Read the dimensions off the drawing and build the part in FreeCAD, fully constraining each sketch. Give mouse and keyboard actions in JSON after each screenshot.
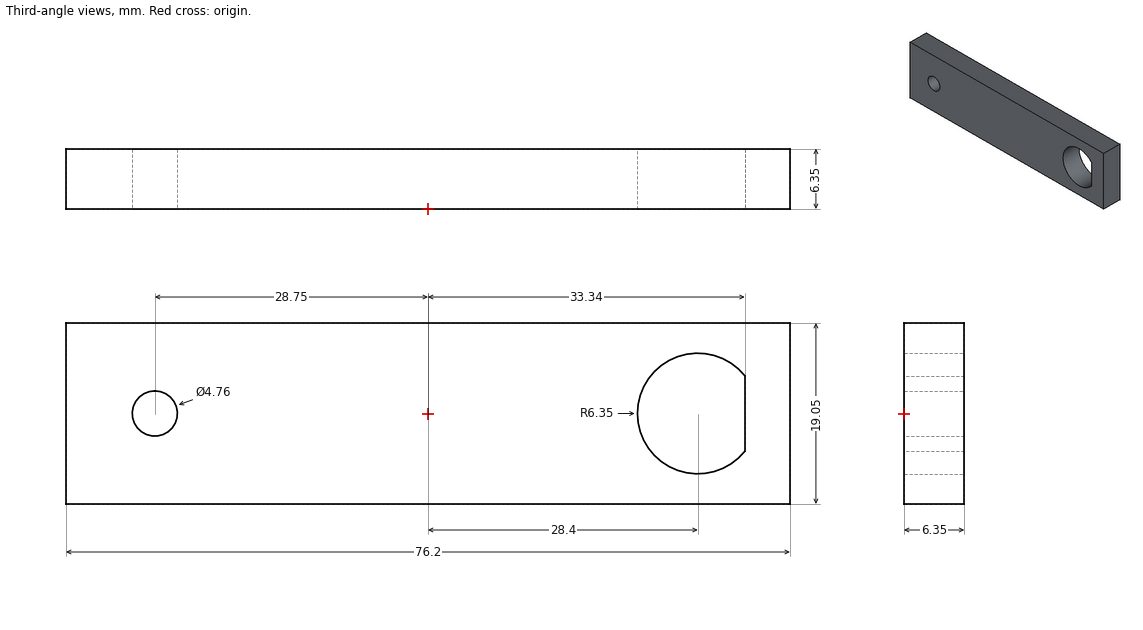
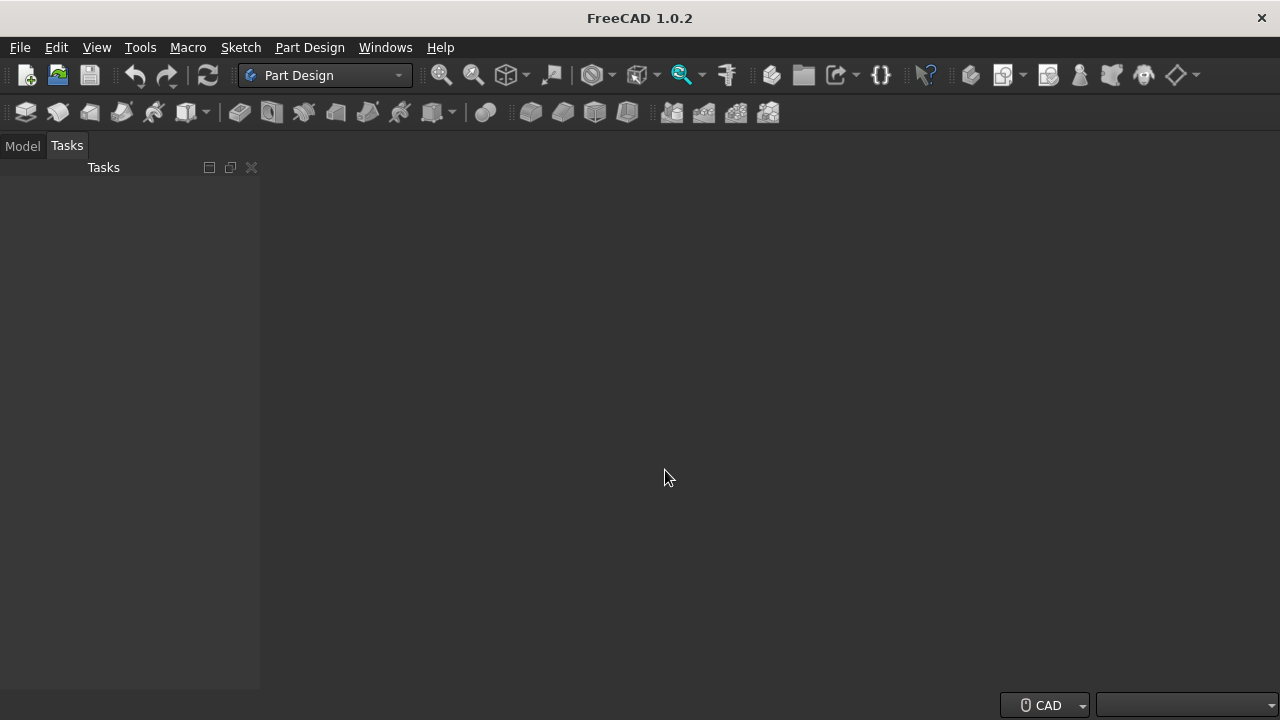
{"action": "key", "text": "ctrl+n"}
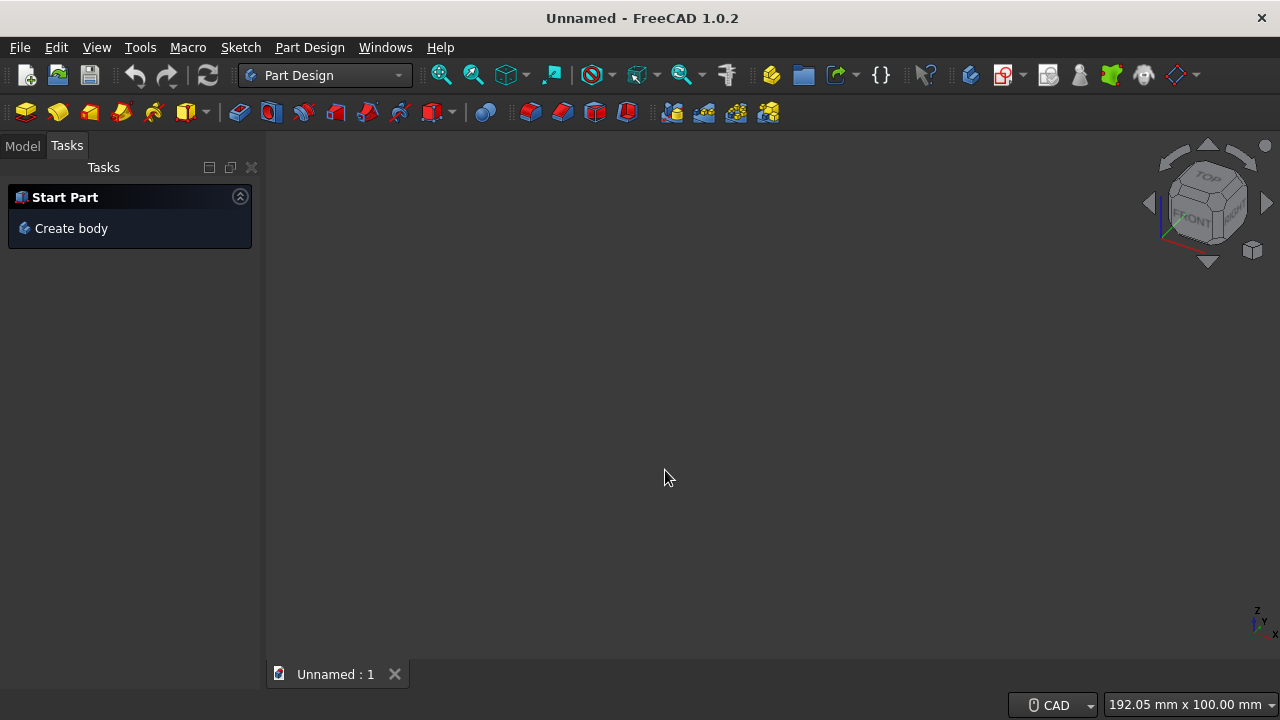
{"action": "left_click", "coordinate": [1004, 76]}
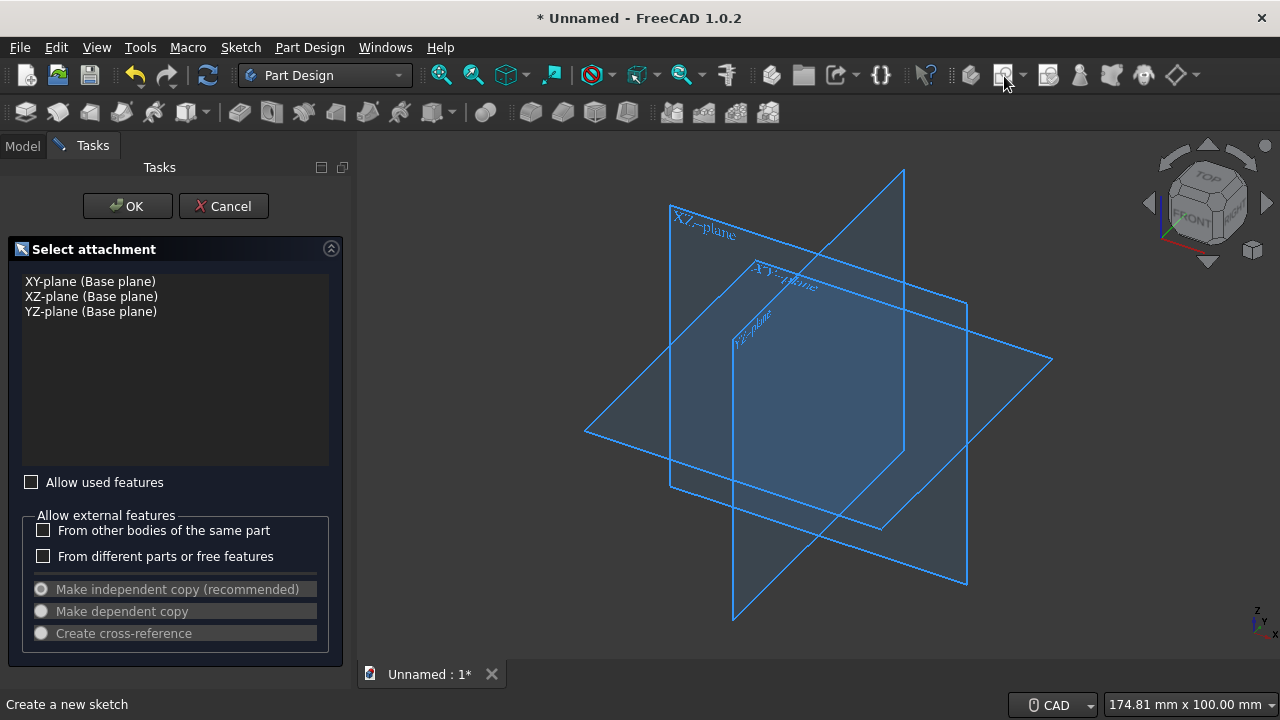
{"action": "left_click", "coordinate": [82, 296]}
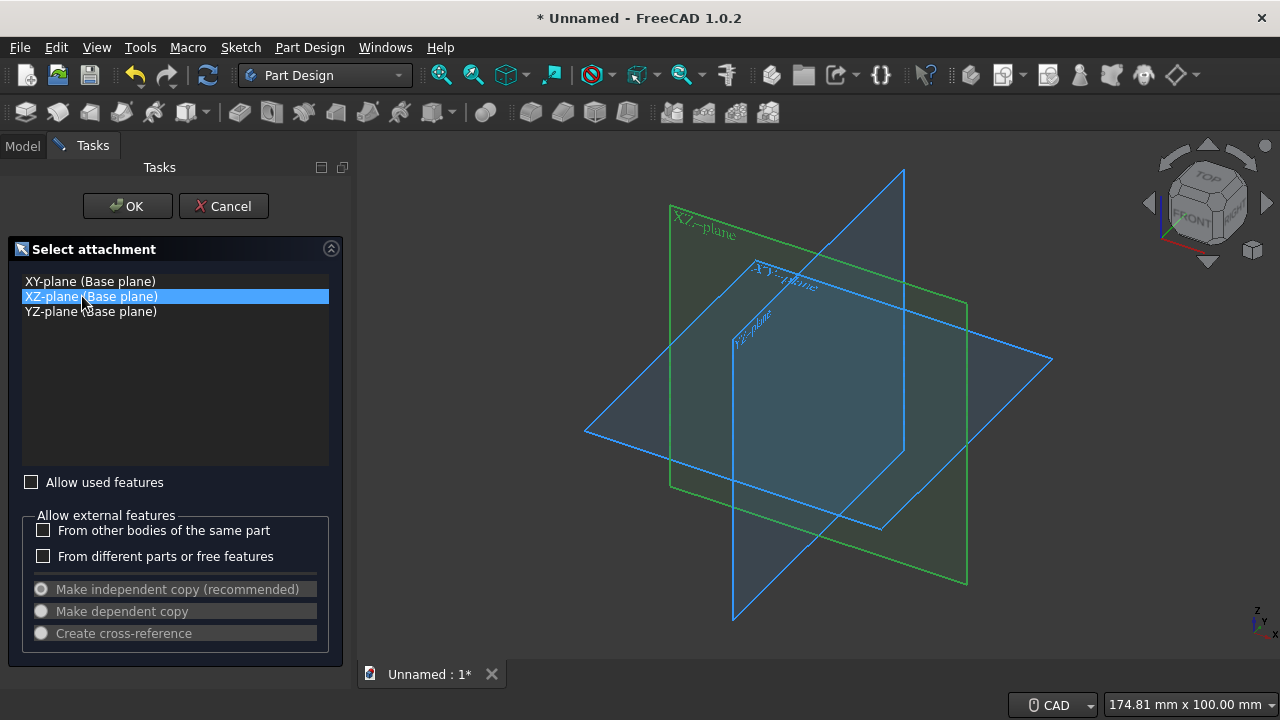
{"action": "left_click", "coordinate": [128, 206]}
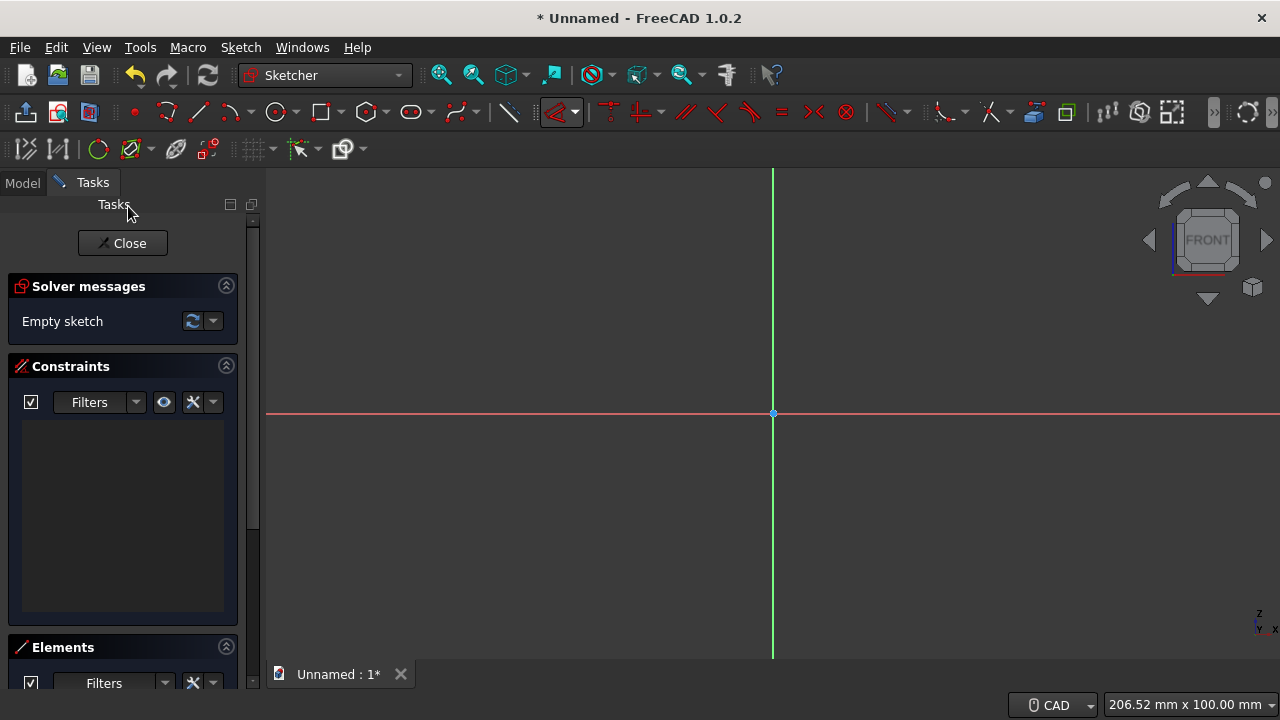
{"action": "scroll", "coordinate": [912, 413], "scroll_direction": "up", "scroll_amount": 2}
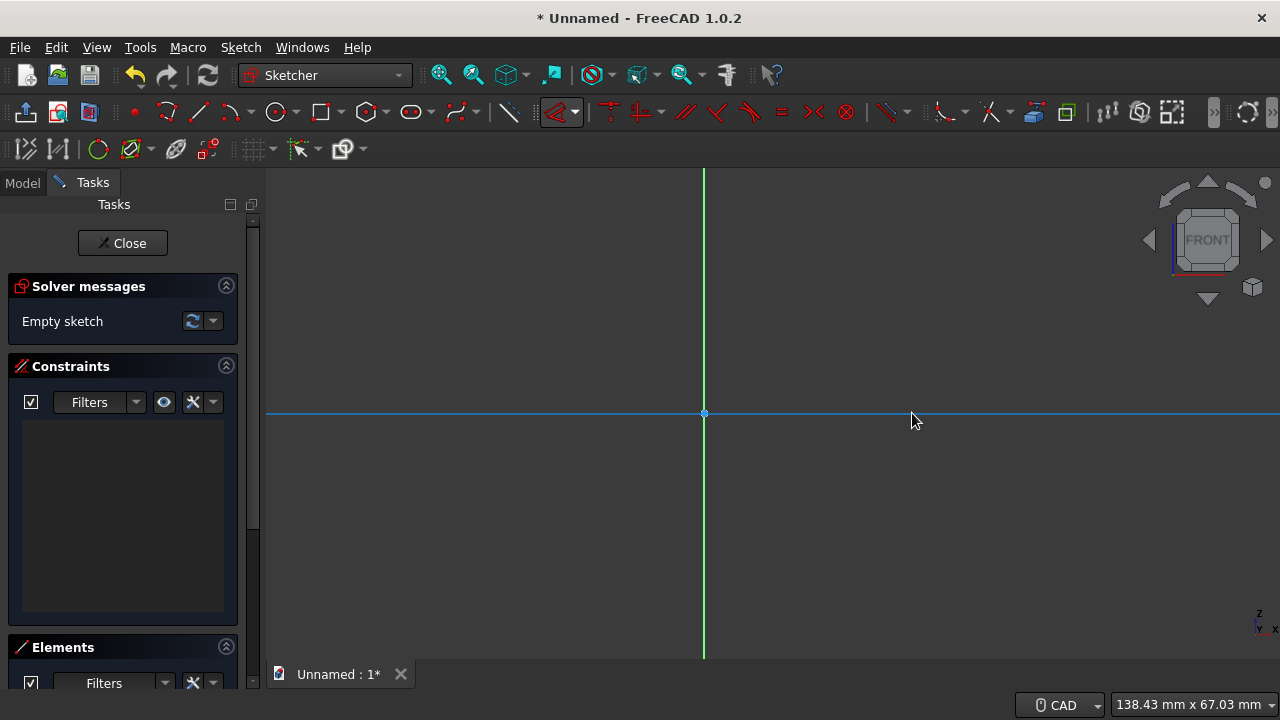
{"action": "key", "text": "g v"}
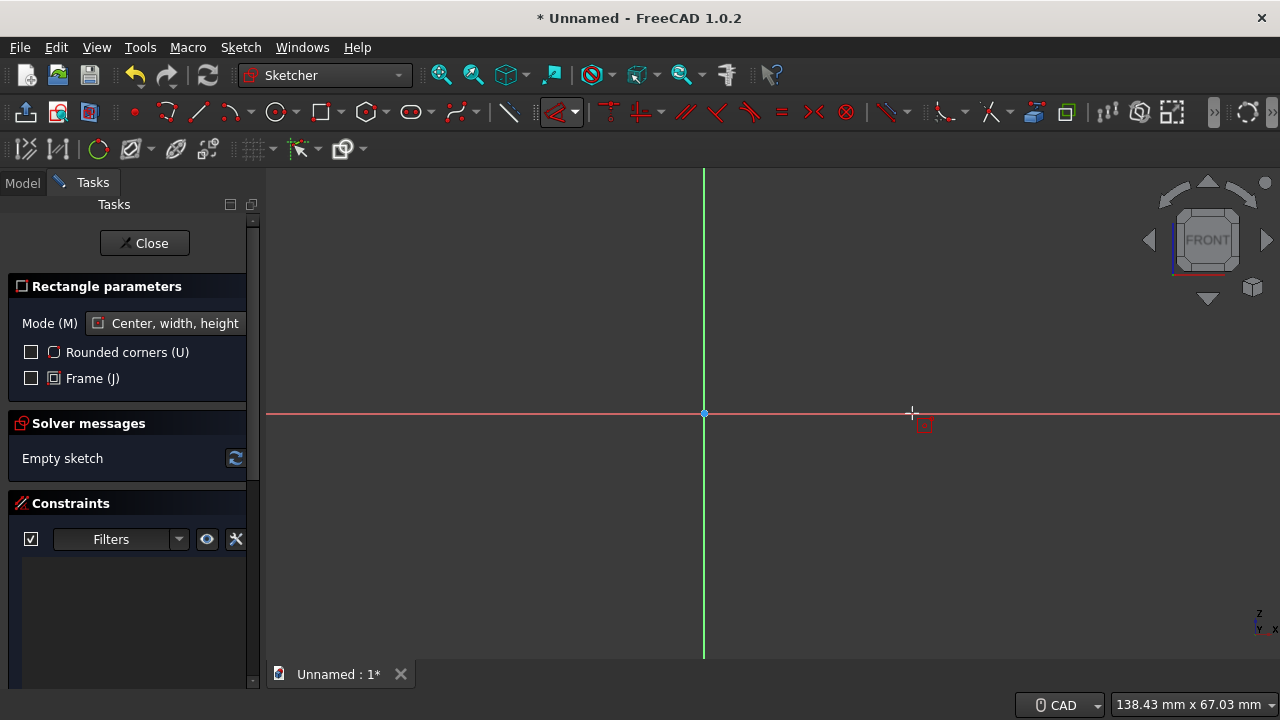
{"action": "left_click", "coordinate": [704, 414]}
{"action": "mouse_move", "coordinate": [983, 344]}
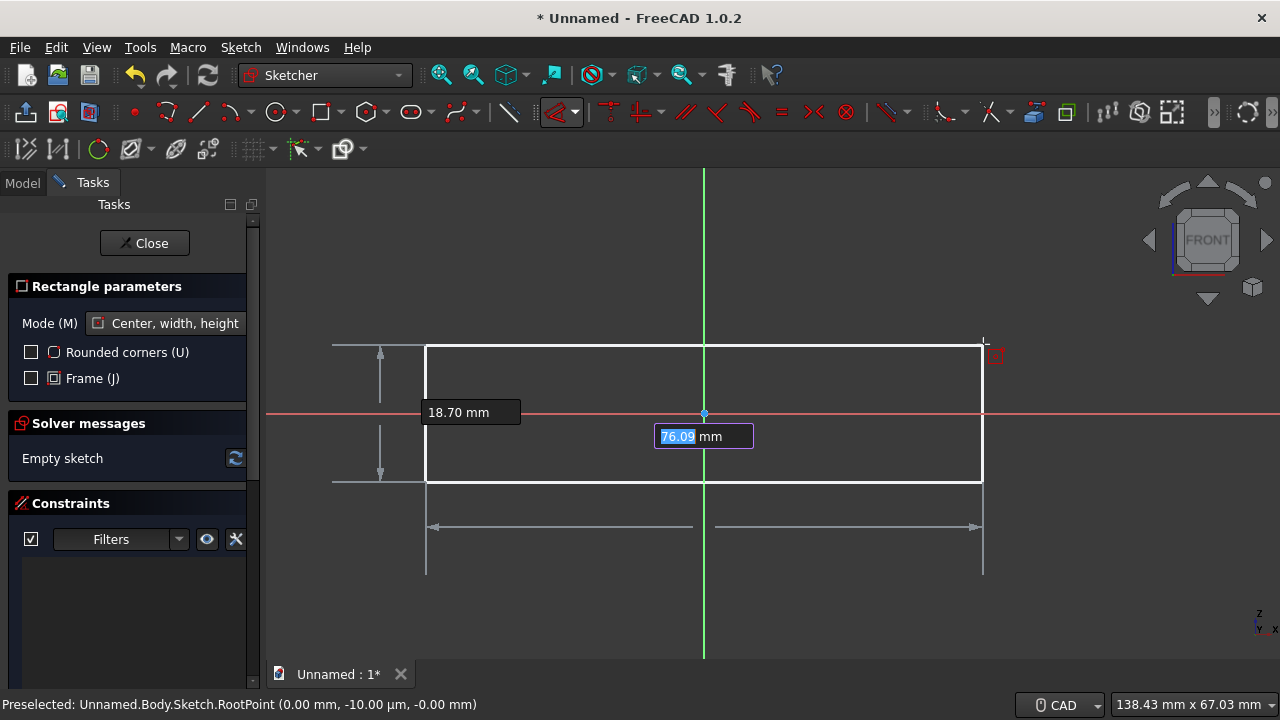
{"action": "type", "text": "76.2"}
{"action": "key", "text": "Tab"}
{"action": "type", "text": "19.05"}
{"action": "key", "text": "Return"}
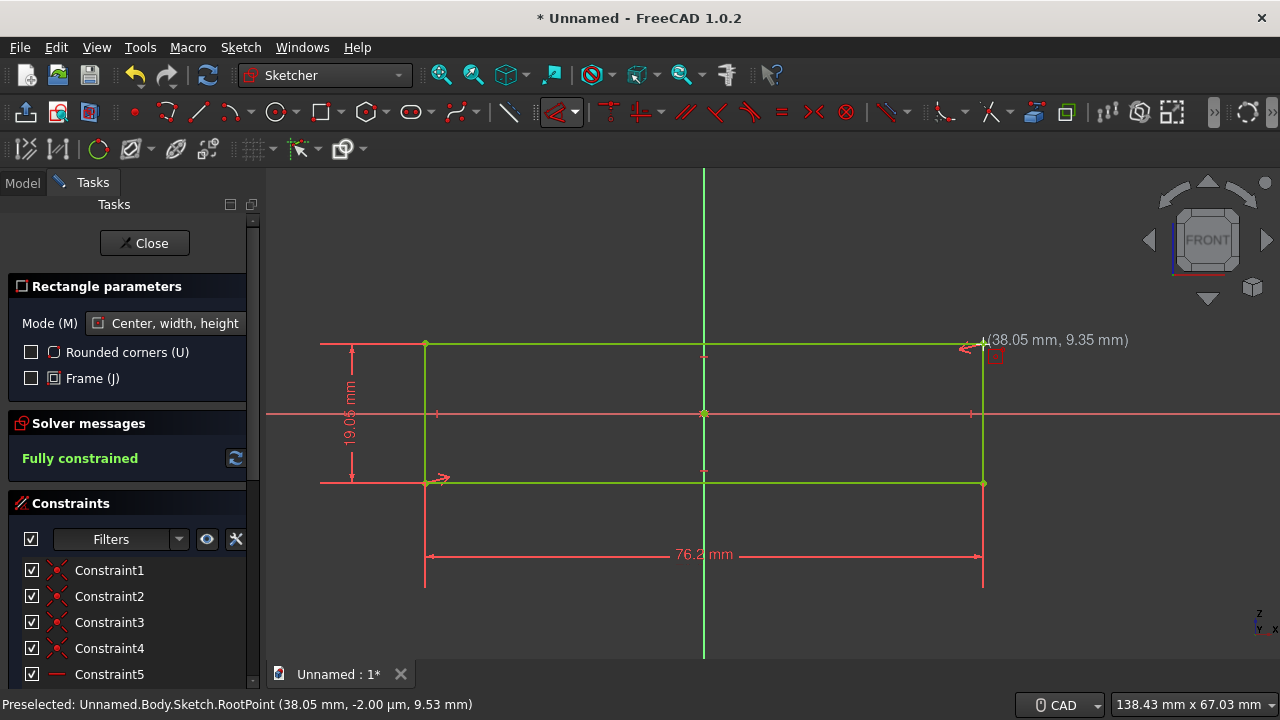
{"action": "key", "text": "g c"}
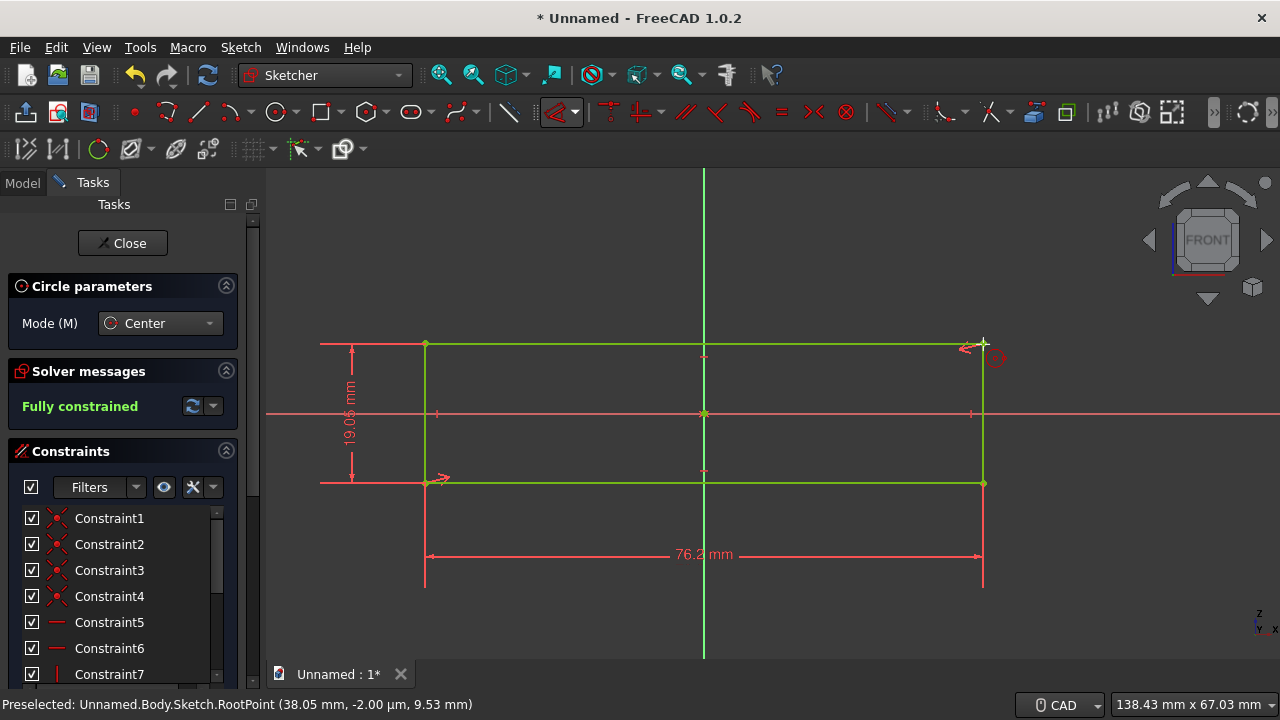
{"action": "scroll", "coordinate": [494, 414], "scroll_direction": "up", "scroll_amount": 2}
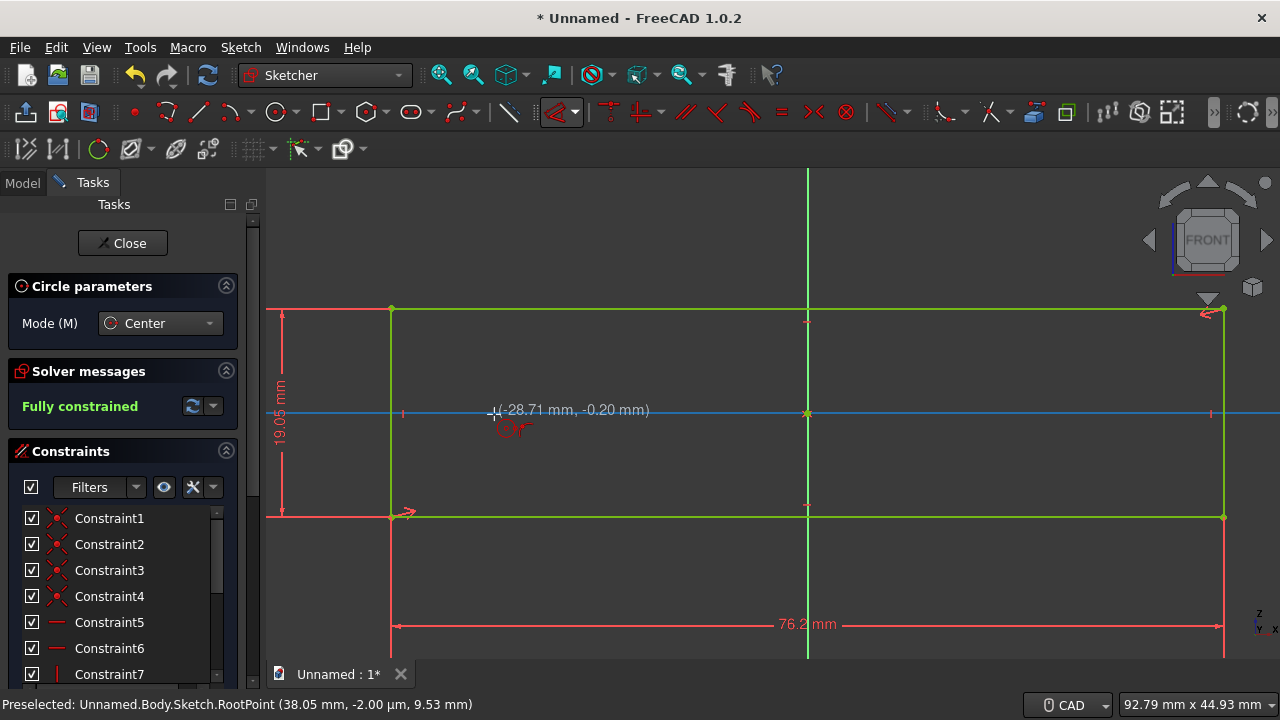
{"action": "left_click", "coordinate": [493, 413]}
{"action": "mouse_move", "coordinate": [512, 395]}